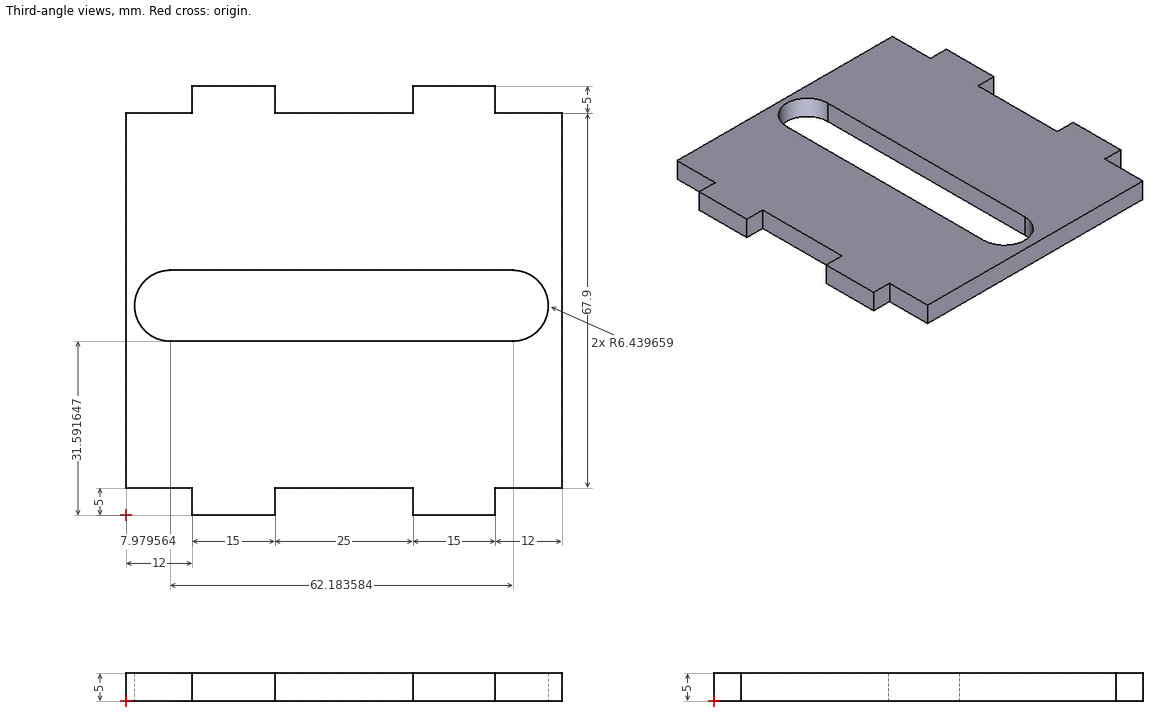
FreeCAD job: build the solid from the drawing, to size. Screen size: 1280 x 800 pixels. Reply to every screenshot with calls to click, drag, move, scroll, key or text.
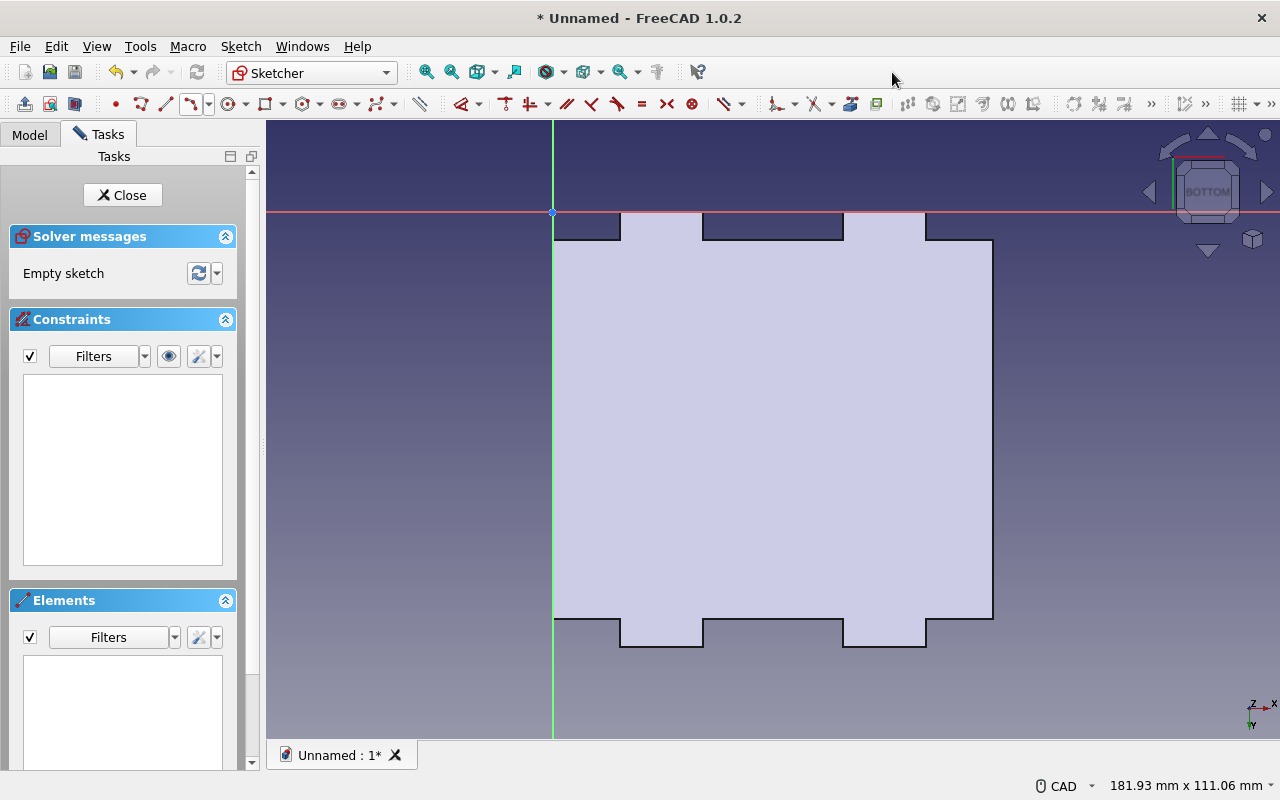
scroll(892, 148, up, 2)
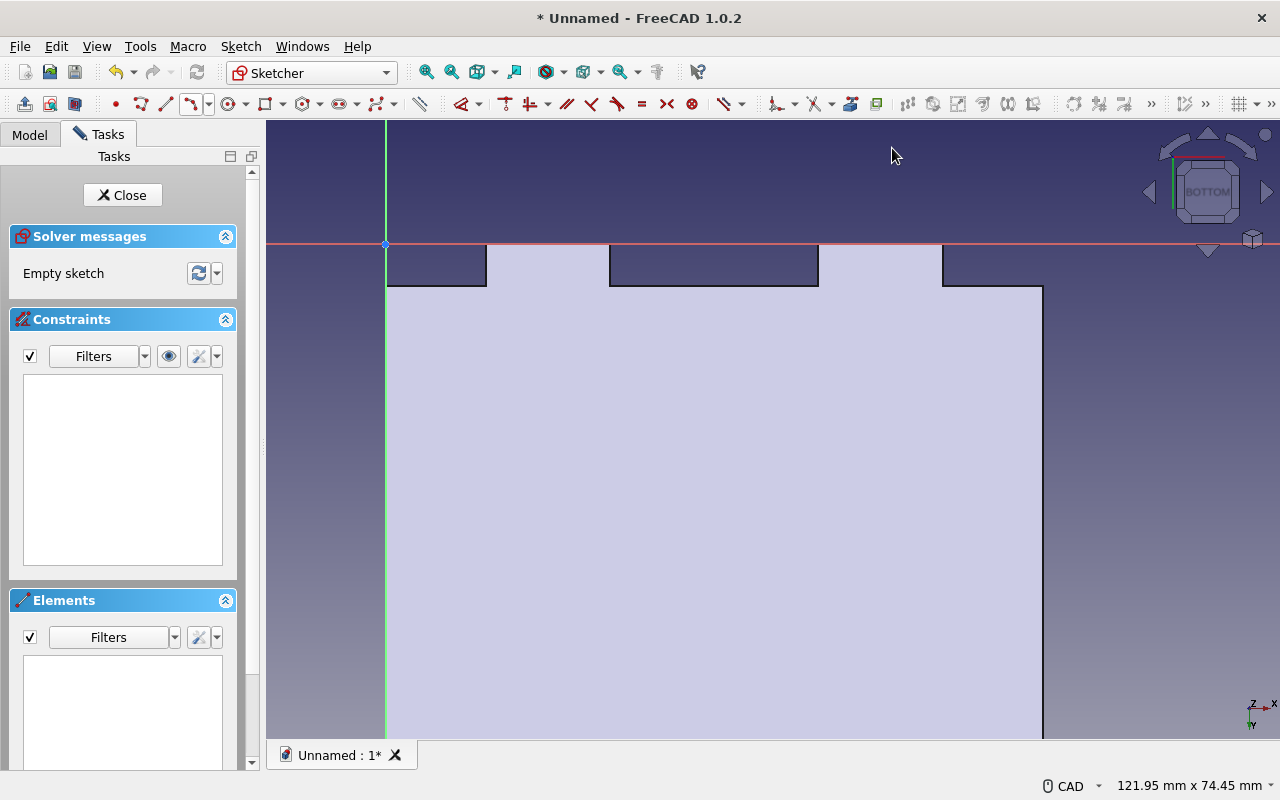
click(338, 104)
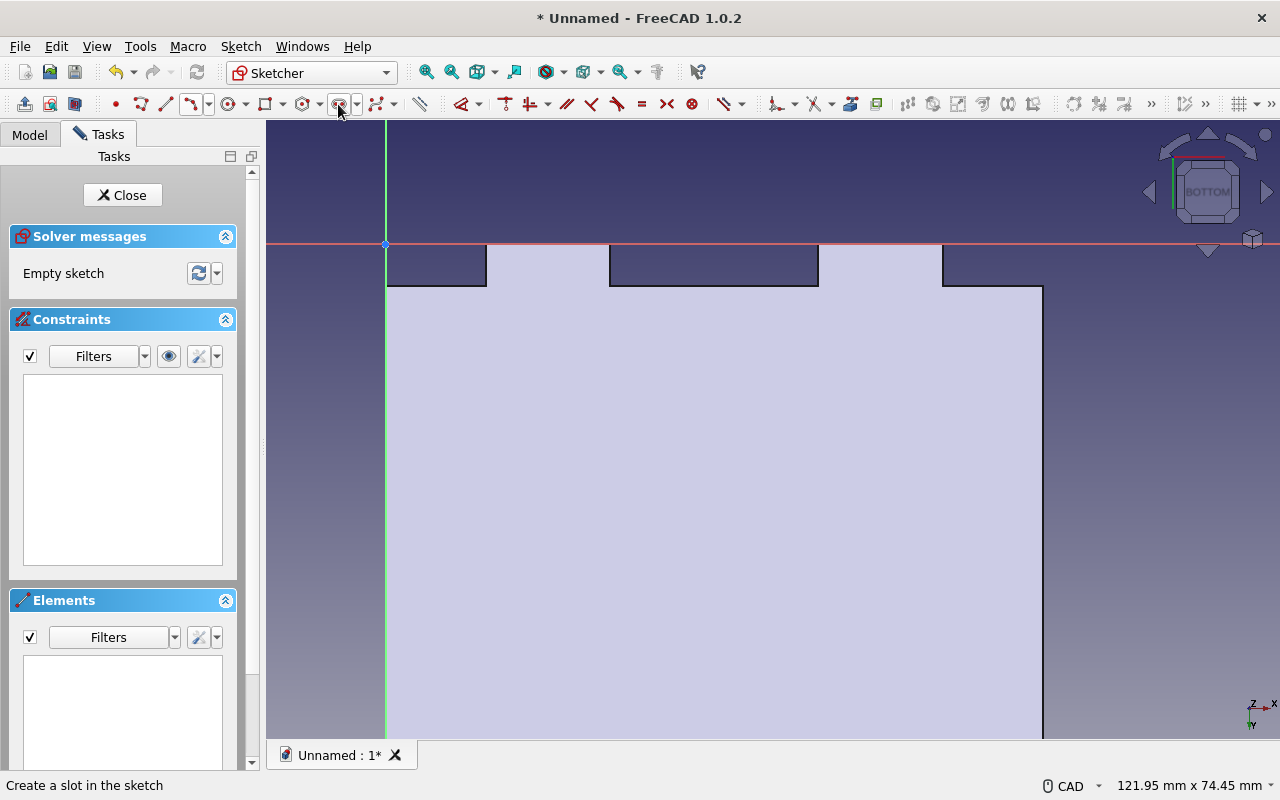
click(452, 560)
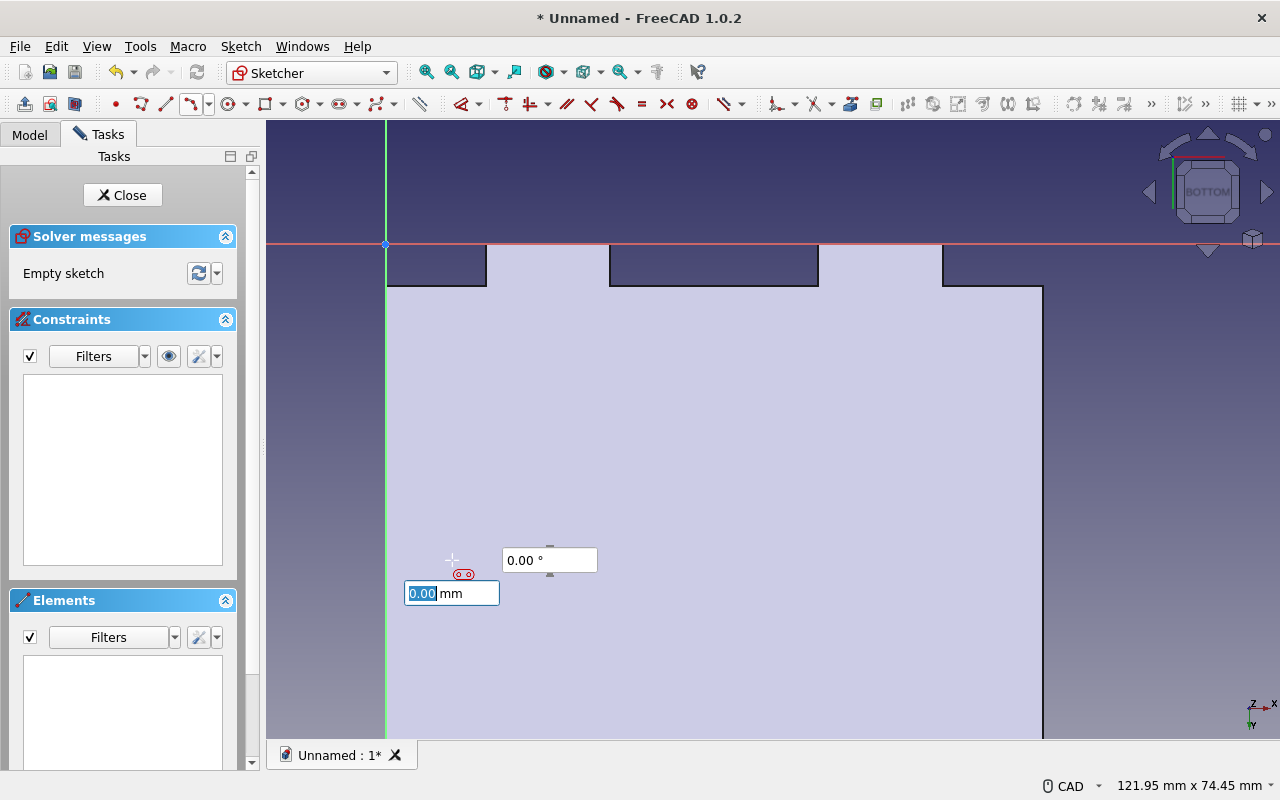
click(969, 560)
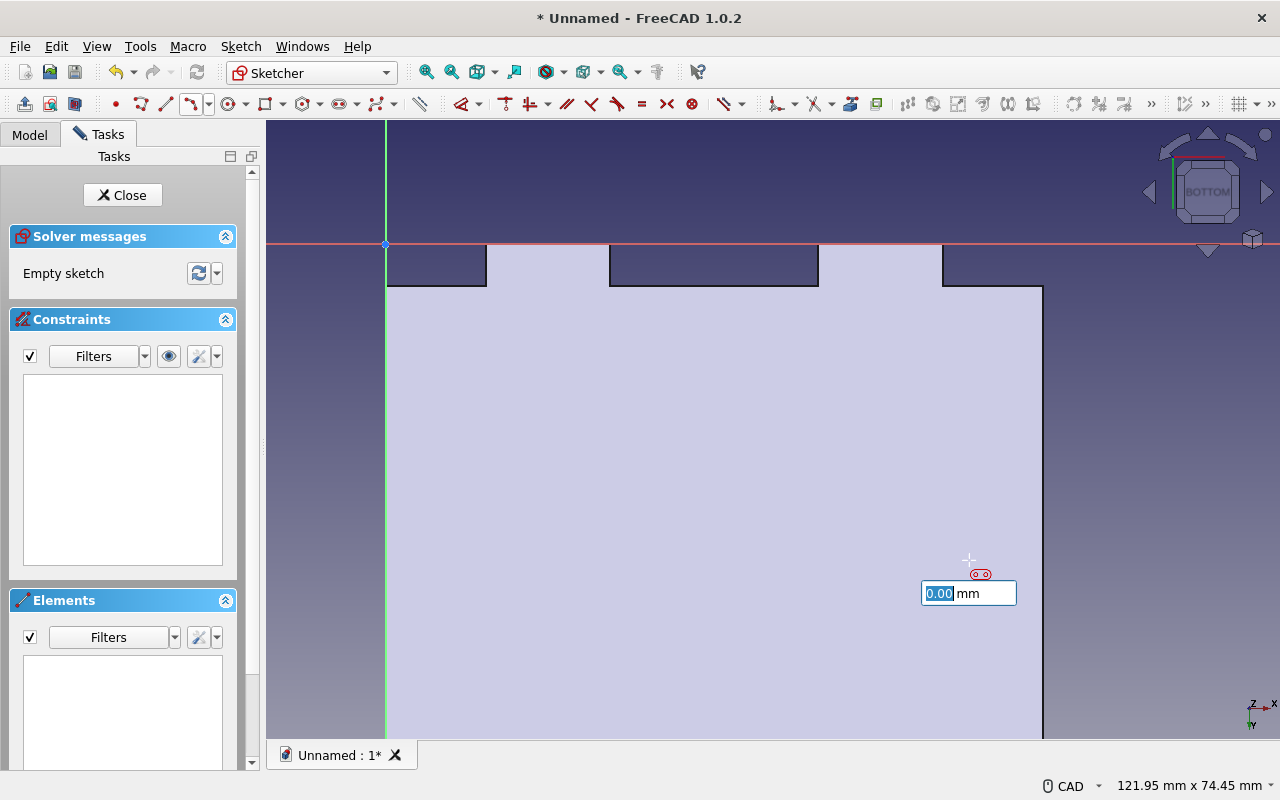
click(711, 614)
key(Escape)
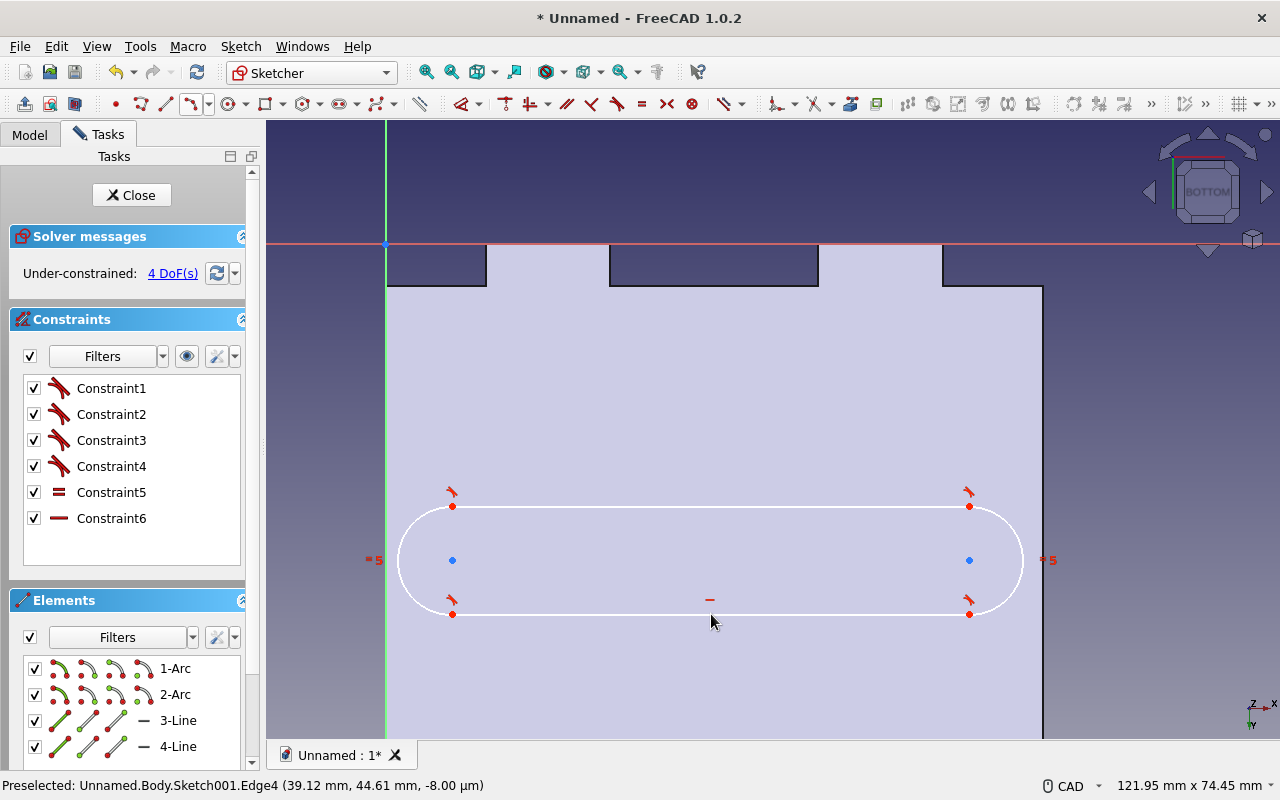
click(460, 104)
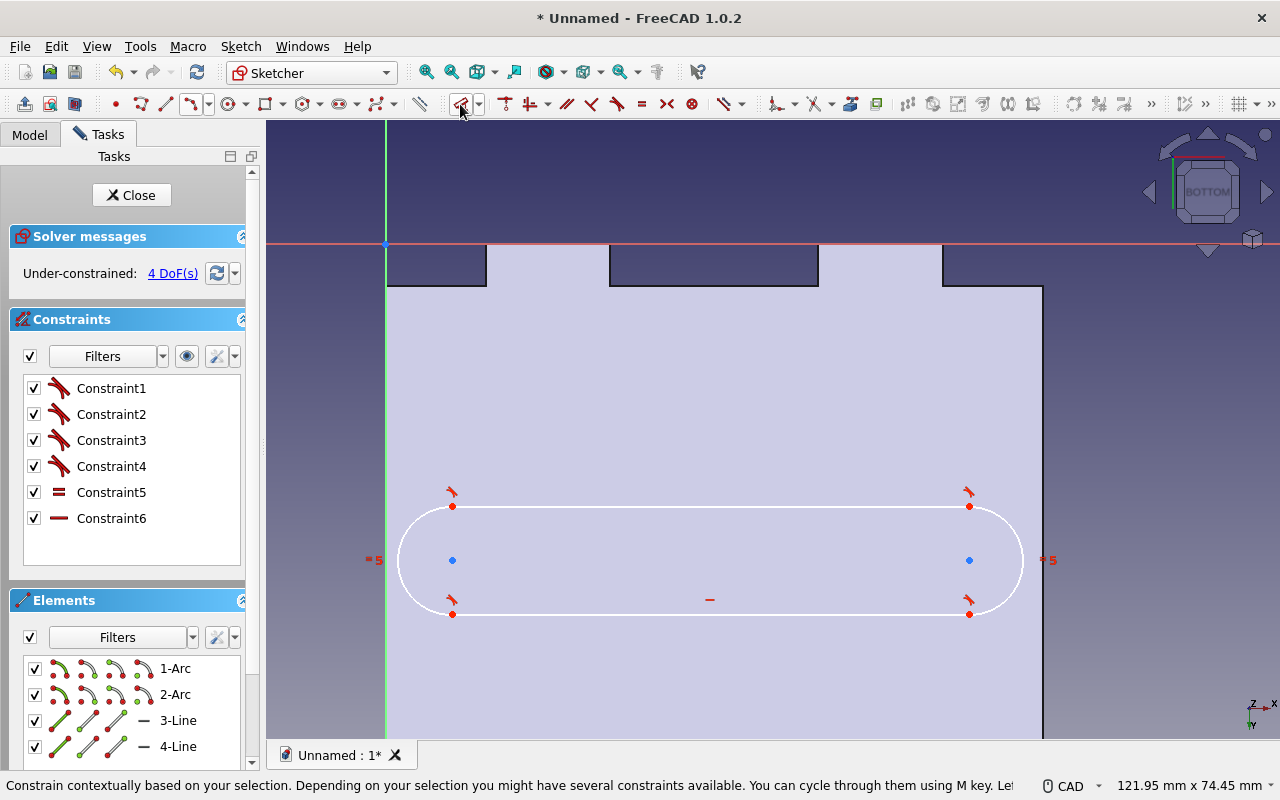
click(408, 529)
click(415, 483)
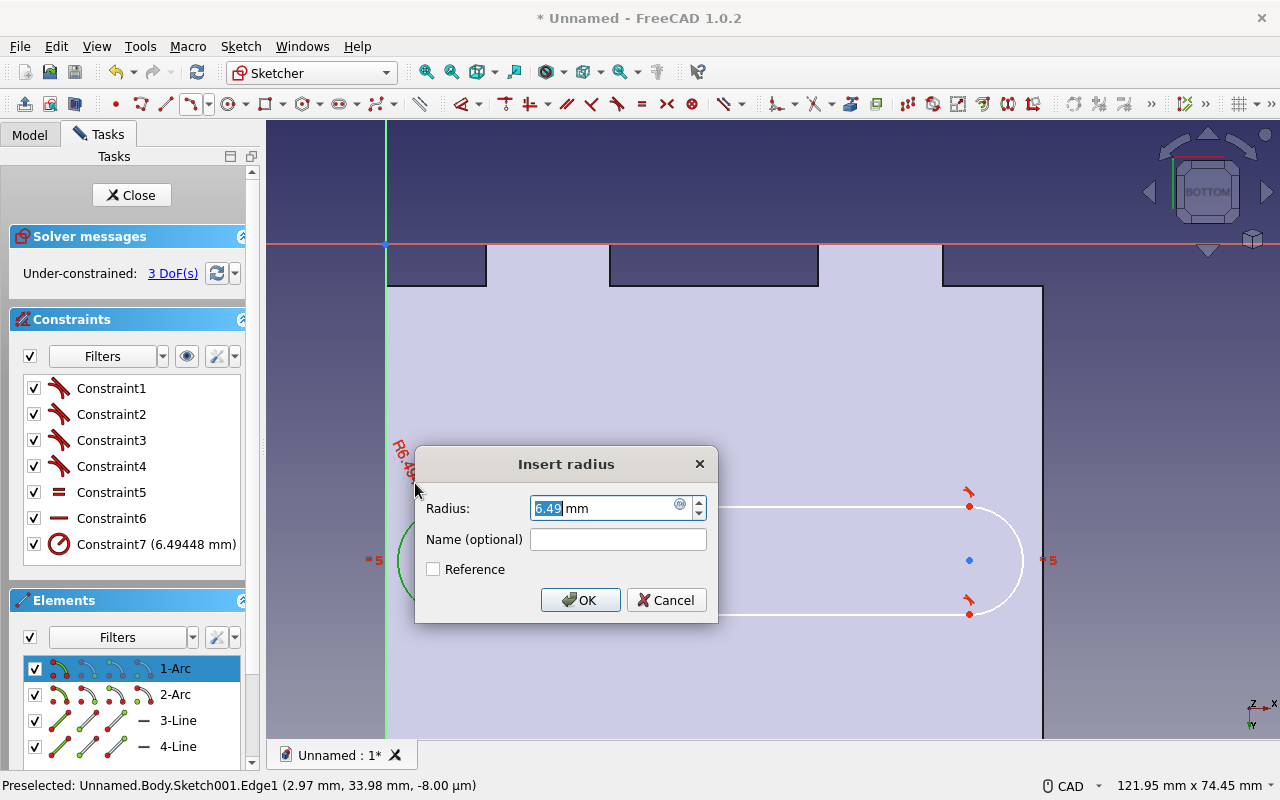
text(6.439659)
key(Return)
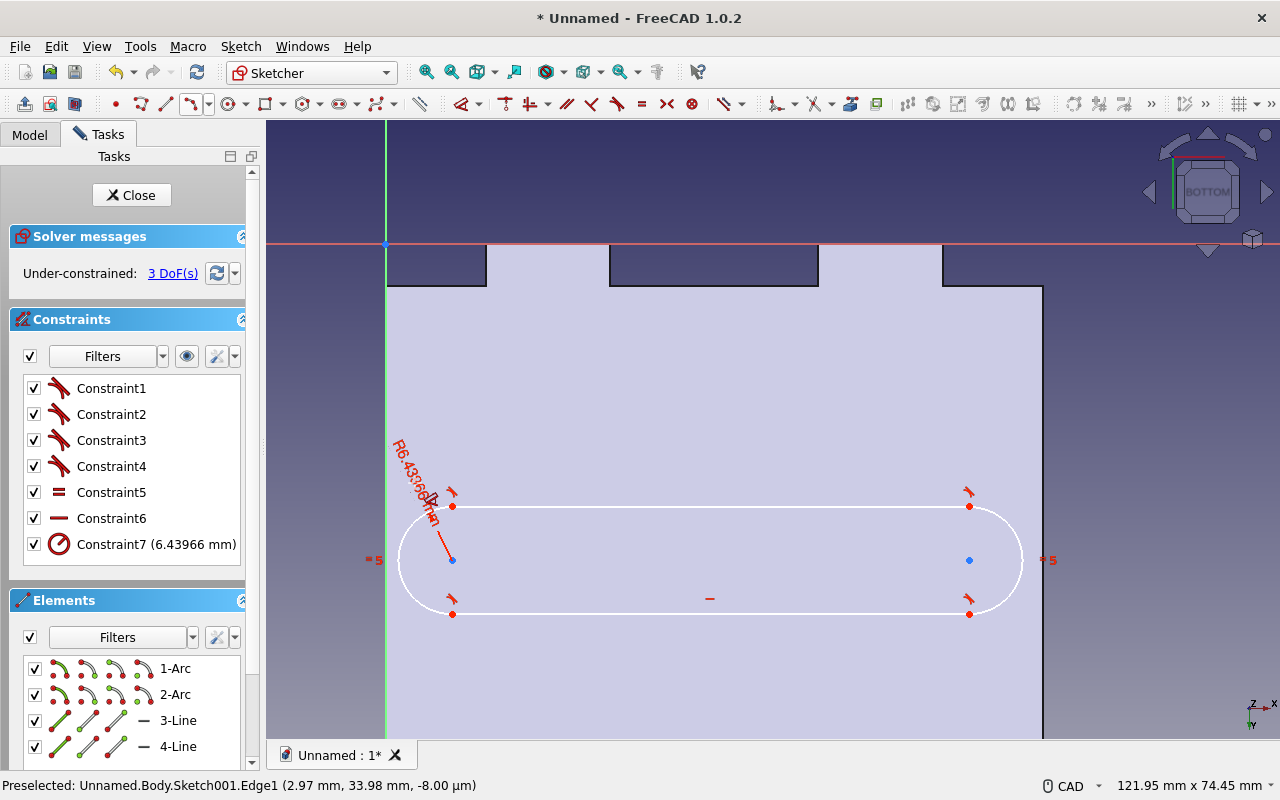
click(607, 507)
click(711, 541)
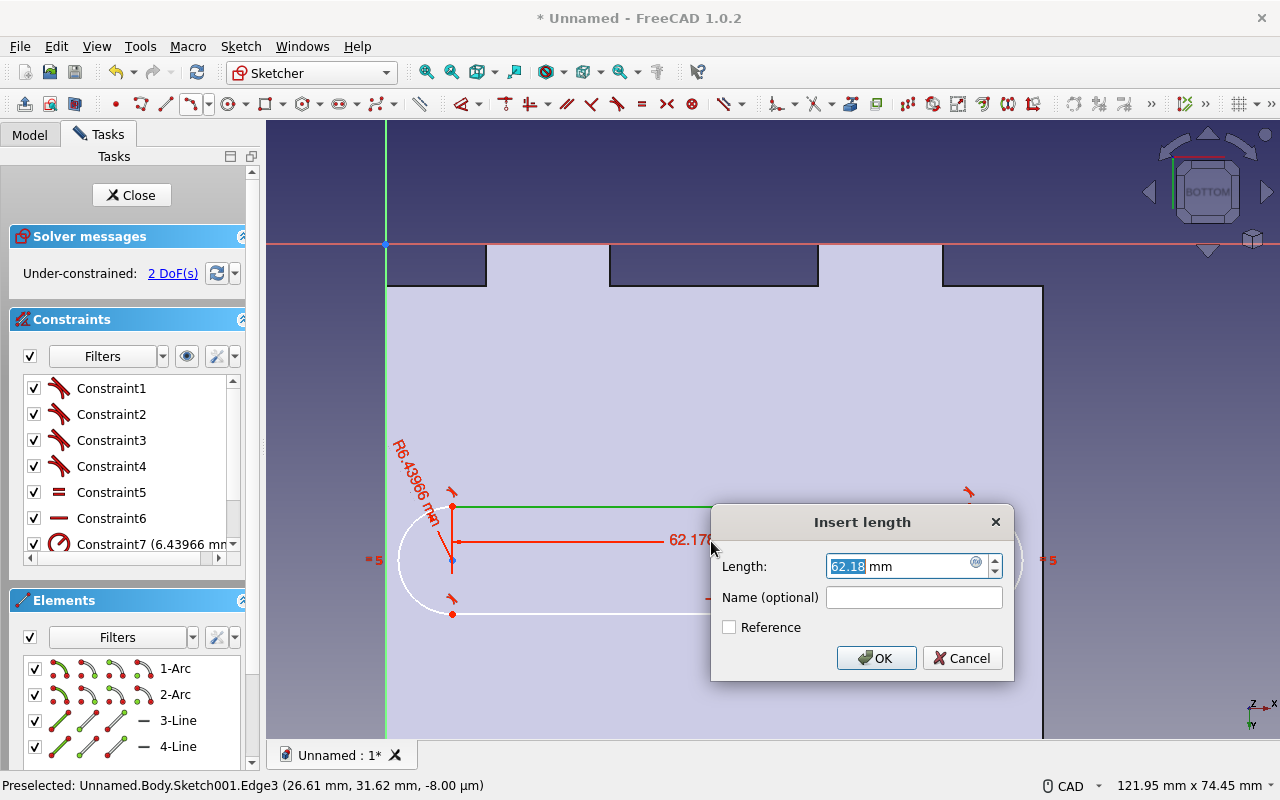
text(62.183584)
key(Return)